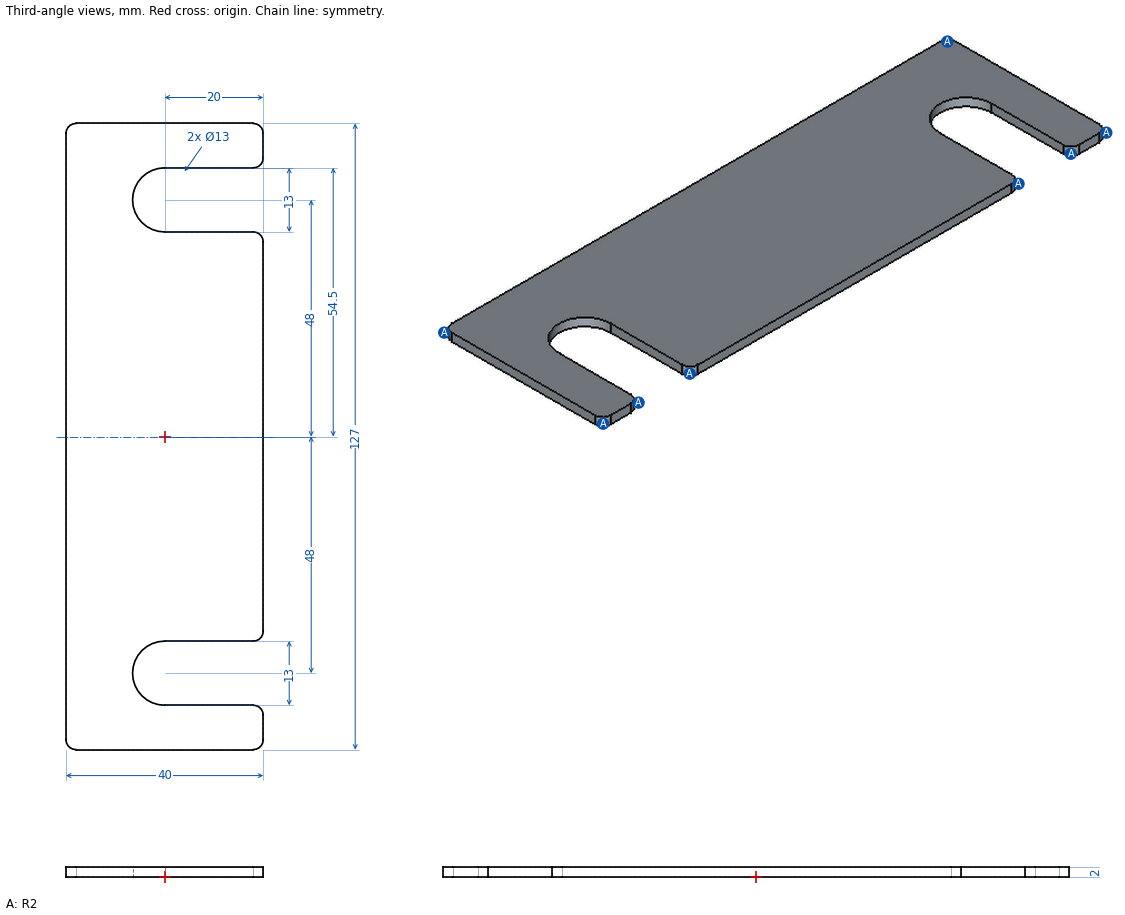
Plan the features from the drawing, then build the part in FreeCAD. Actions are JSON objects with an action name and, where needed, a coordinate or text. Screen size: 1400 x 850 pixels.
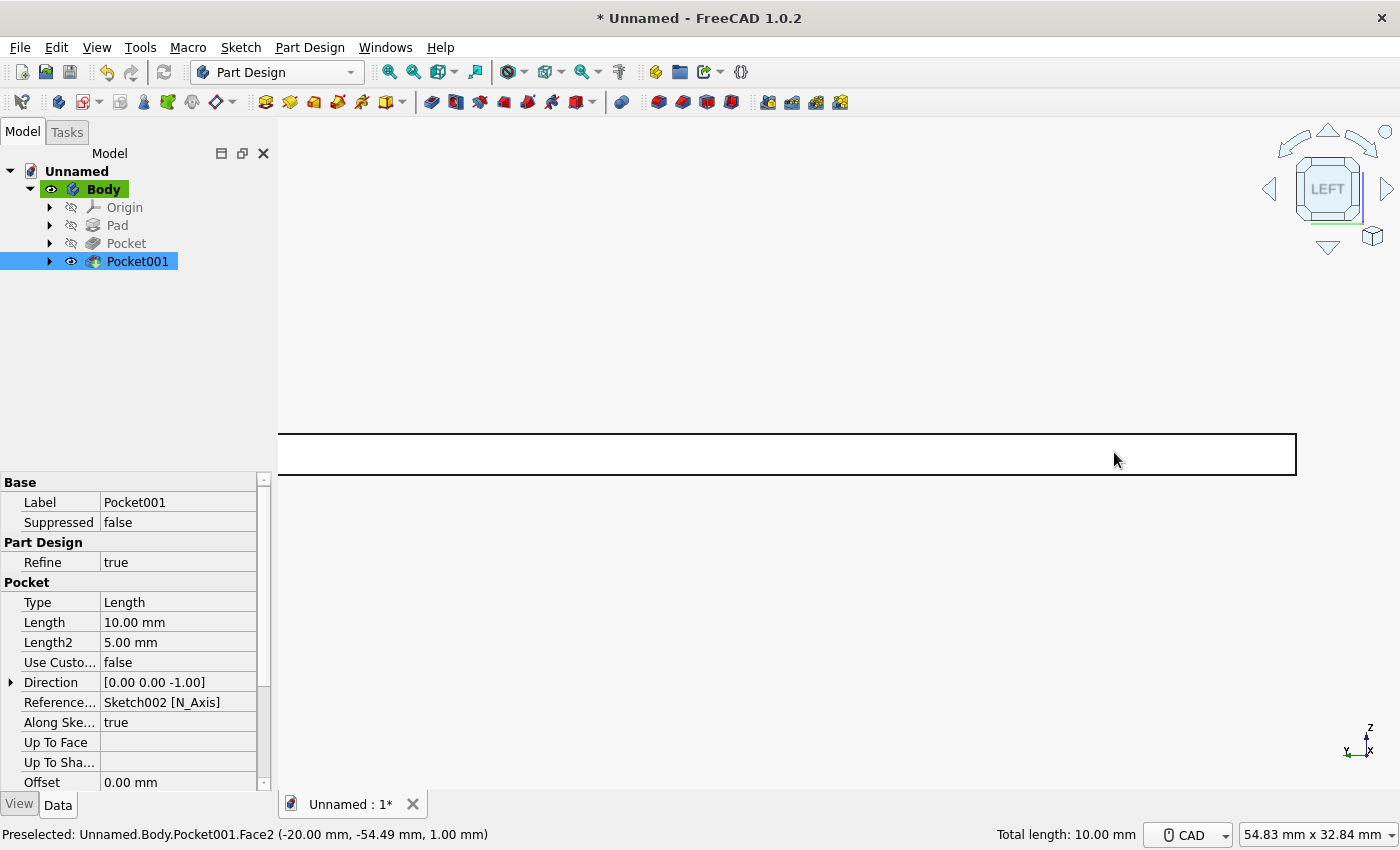
{"action": "left_click", "coordinate": [1296, 454], "text": "ctrl"}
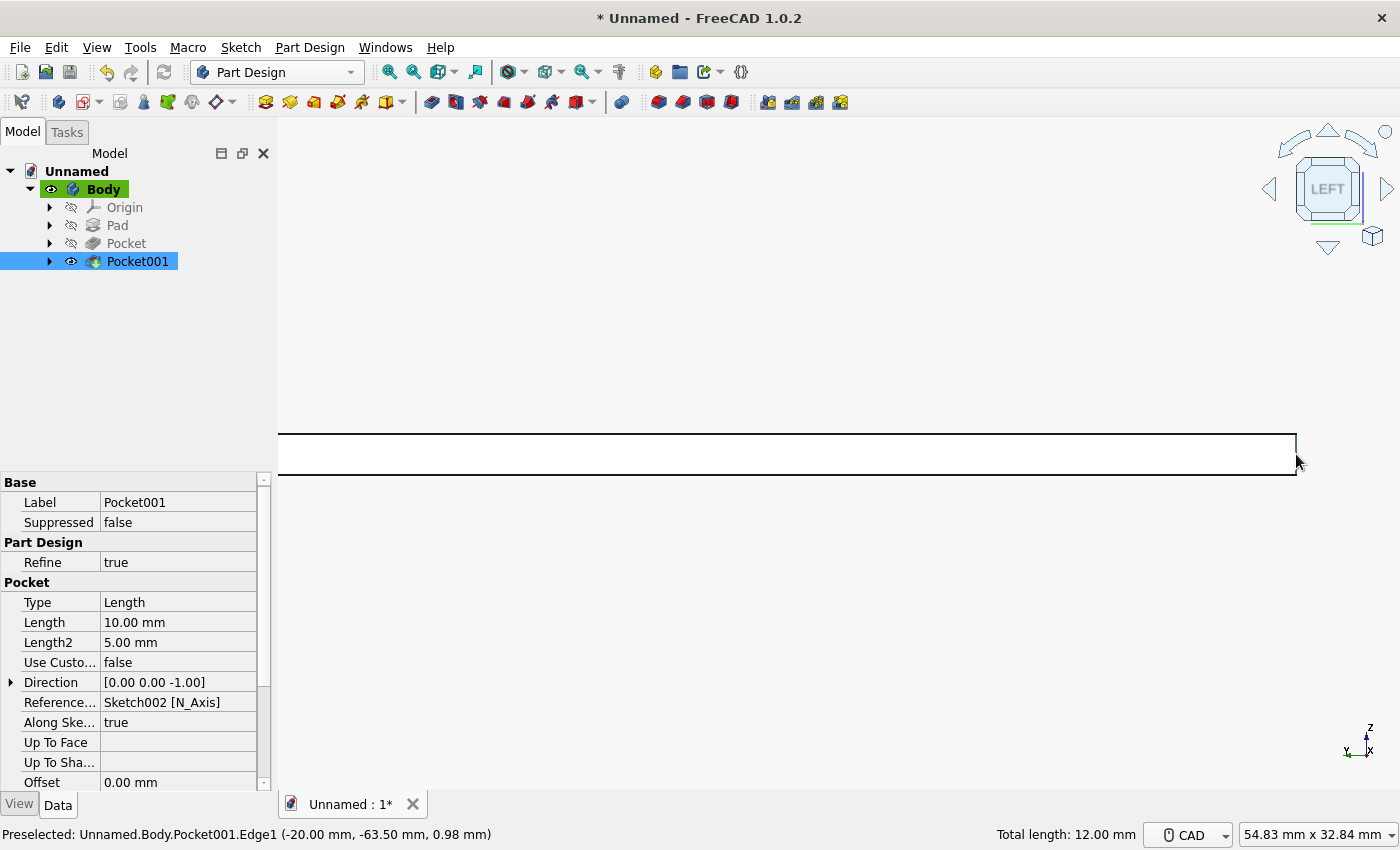
{"action": "left_click", "coordinate": [390, 72]}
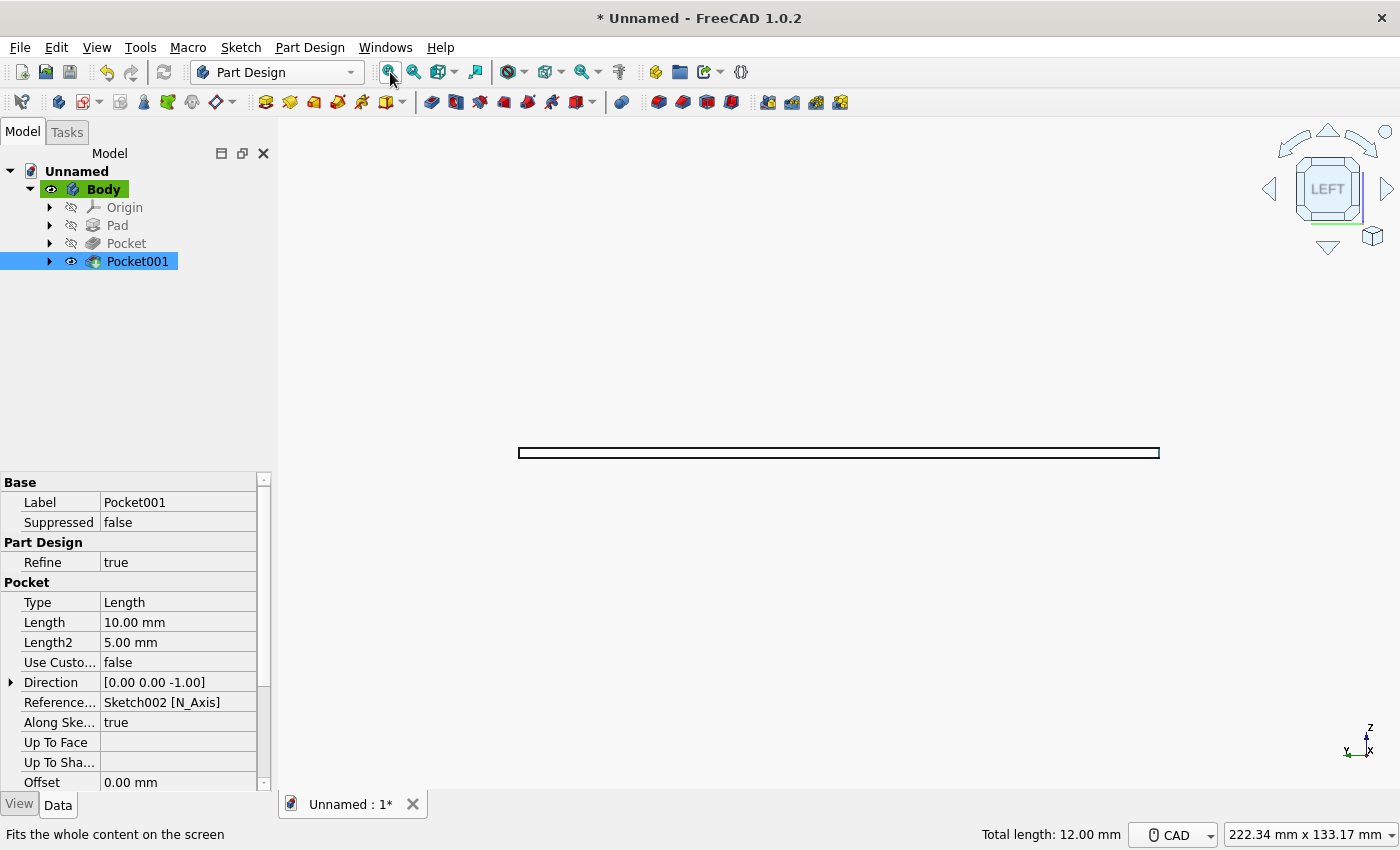
{"action": "key", "text": "v 3"}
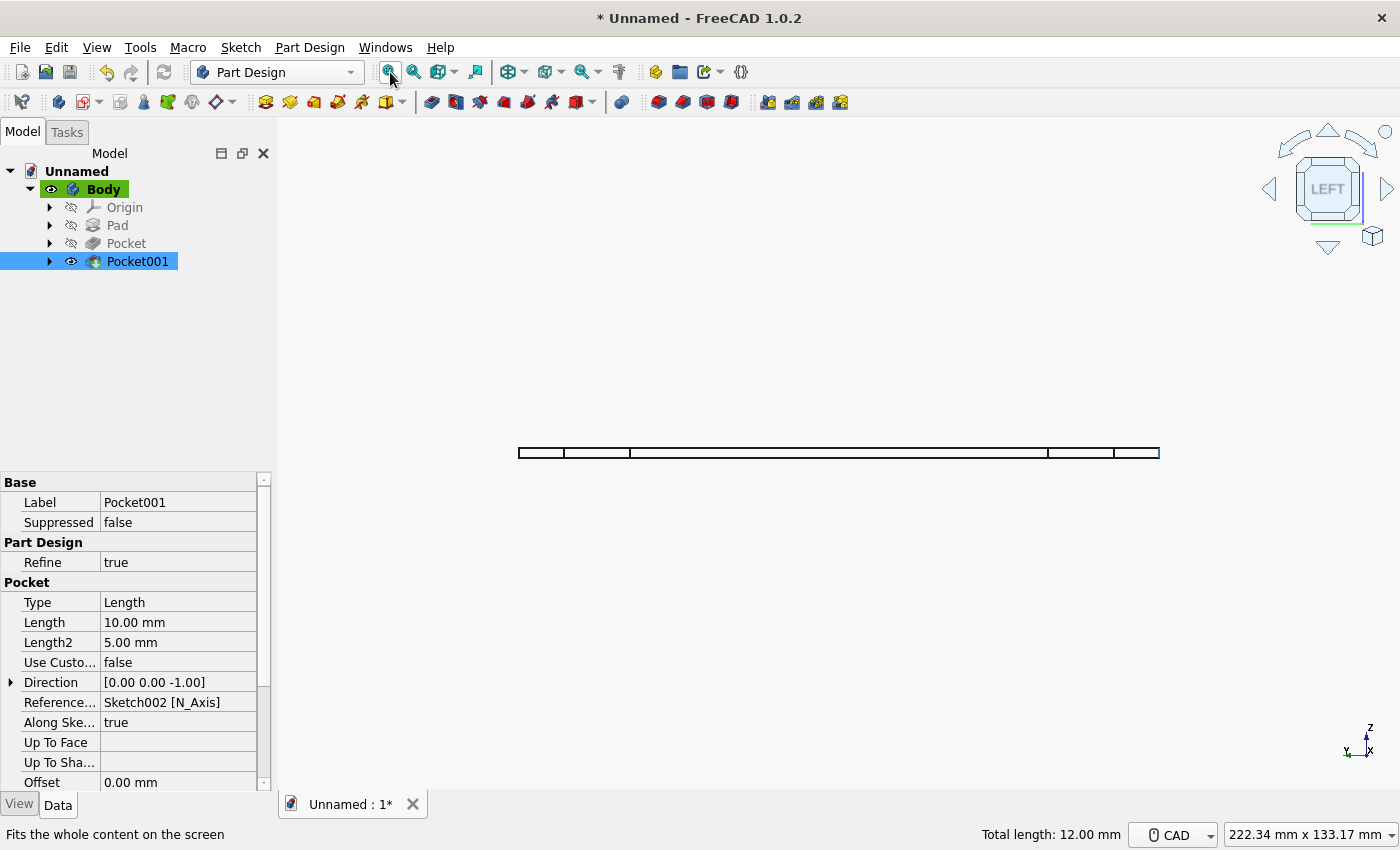
{"action": "key", "text": "0"}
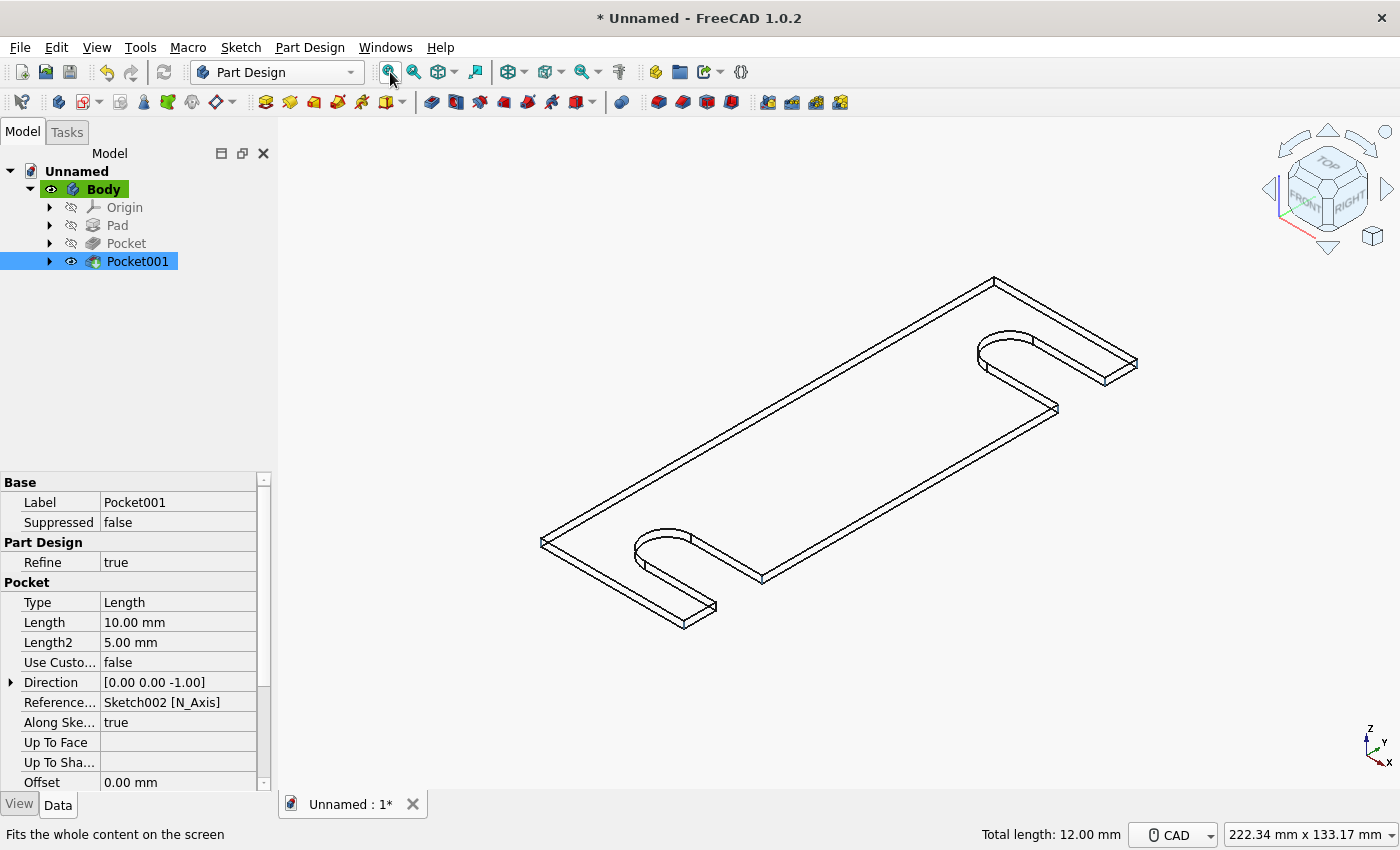
{"action": "scroll", "coordinate": [716, 605], "scroll_direction": "up", "scroll_amount": 7}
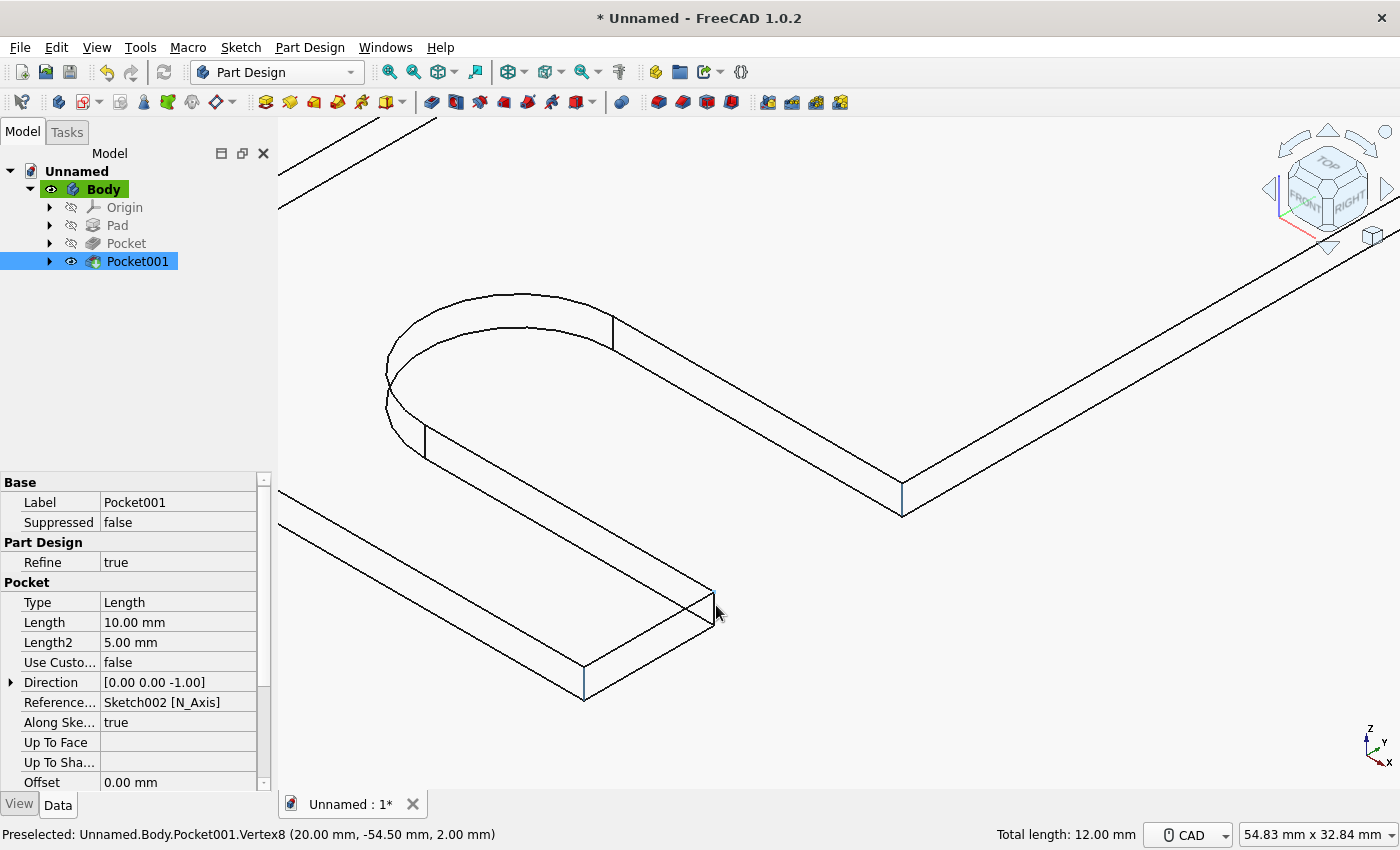
{"action": "left_click", "coordinate": [714, 608], "text": "ctrl"}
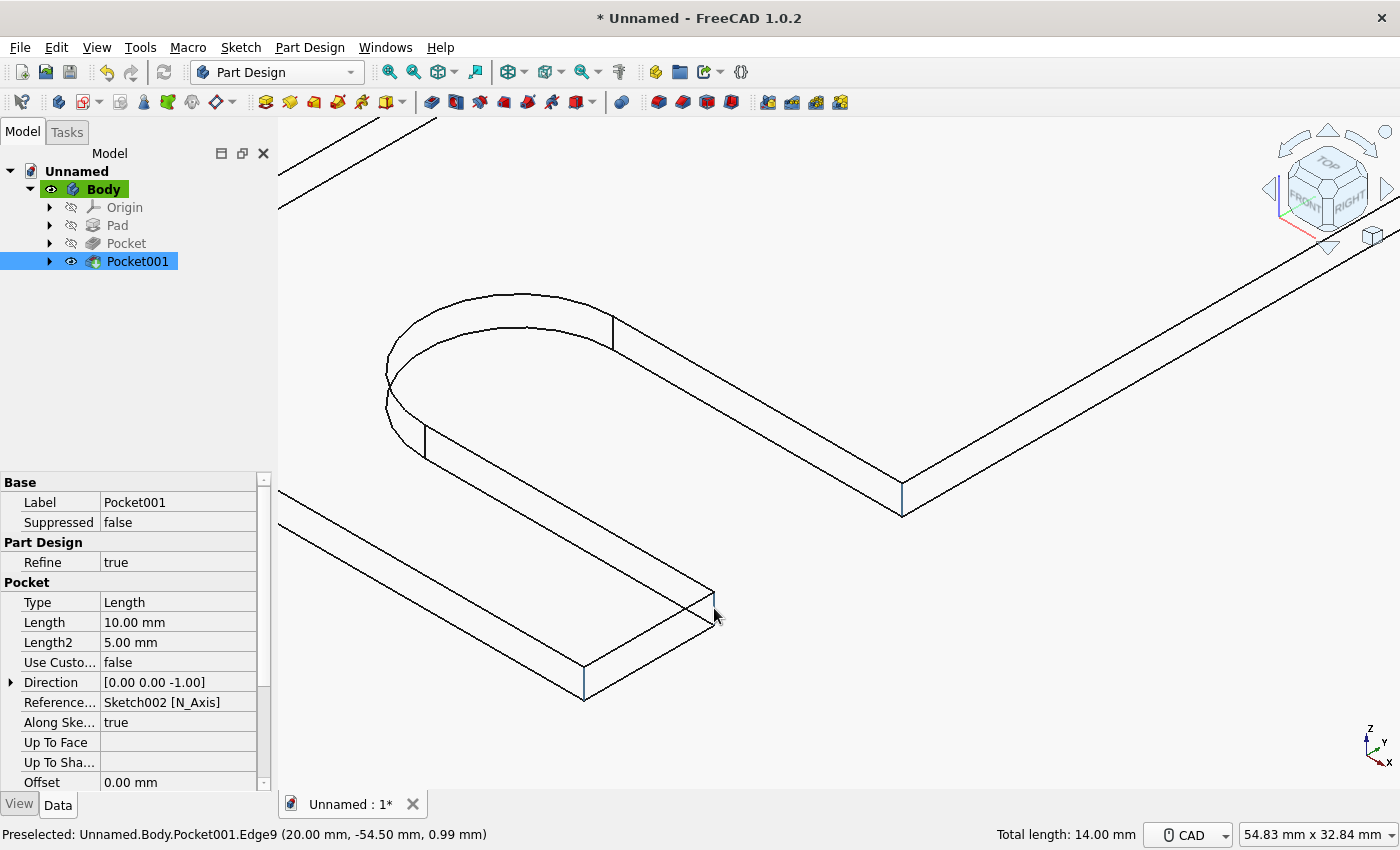
{"action": "left_click", "coordinate": [390, 72]}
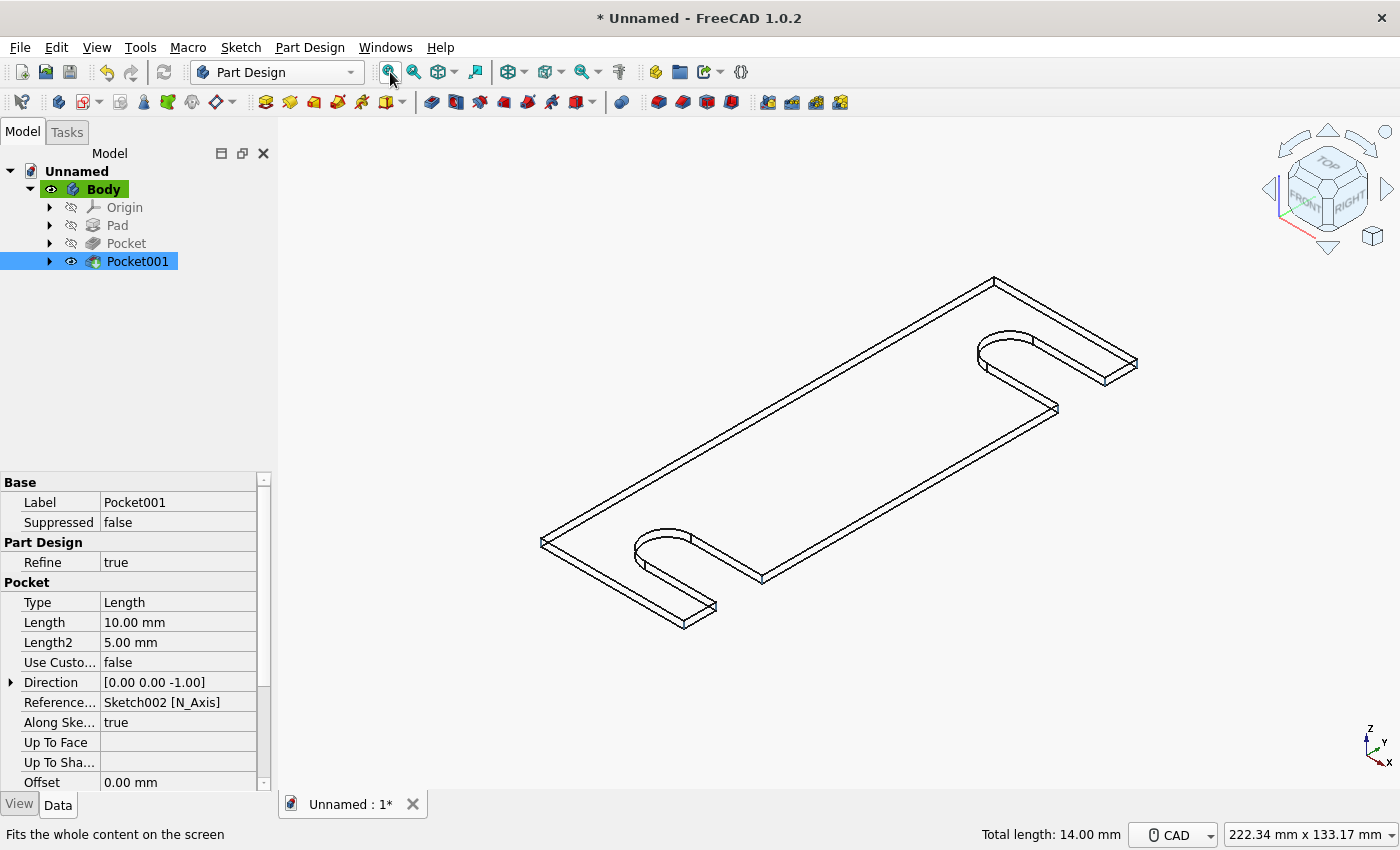
{"action": "key", "text": "2"}